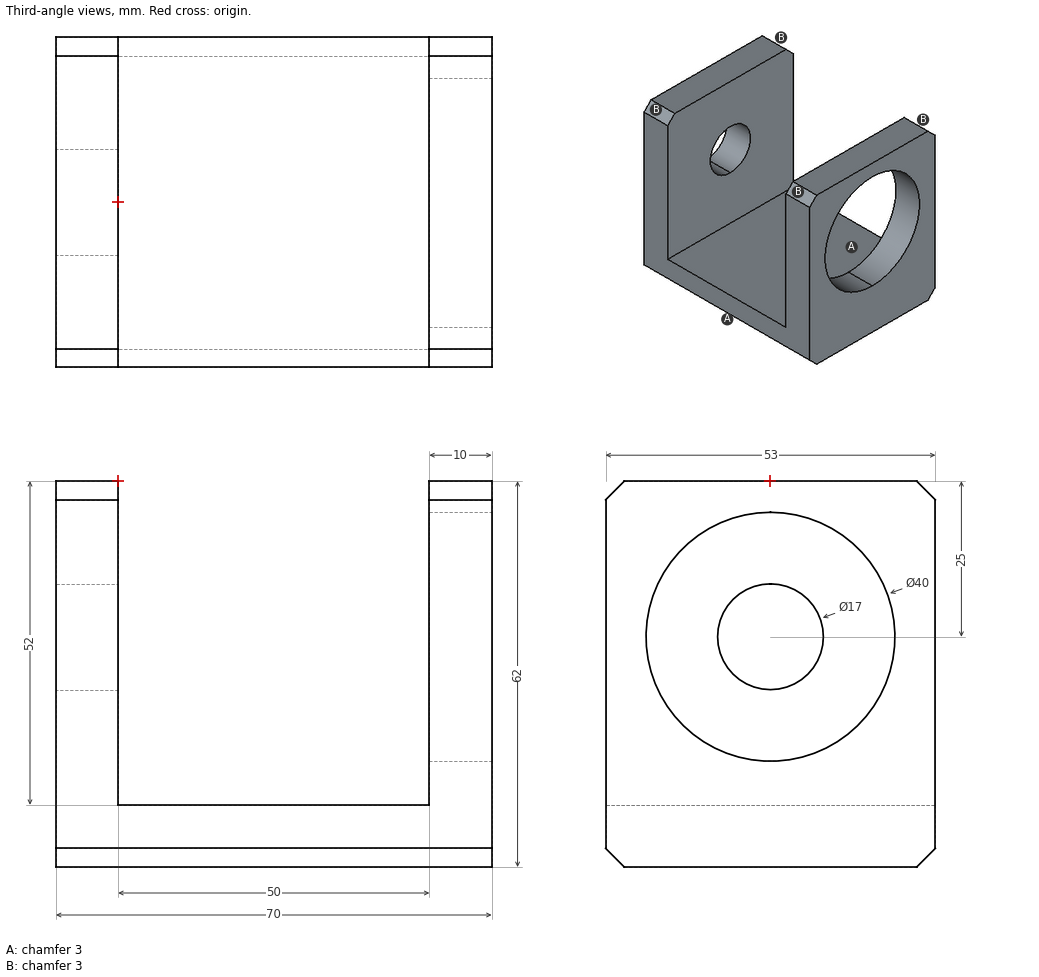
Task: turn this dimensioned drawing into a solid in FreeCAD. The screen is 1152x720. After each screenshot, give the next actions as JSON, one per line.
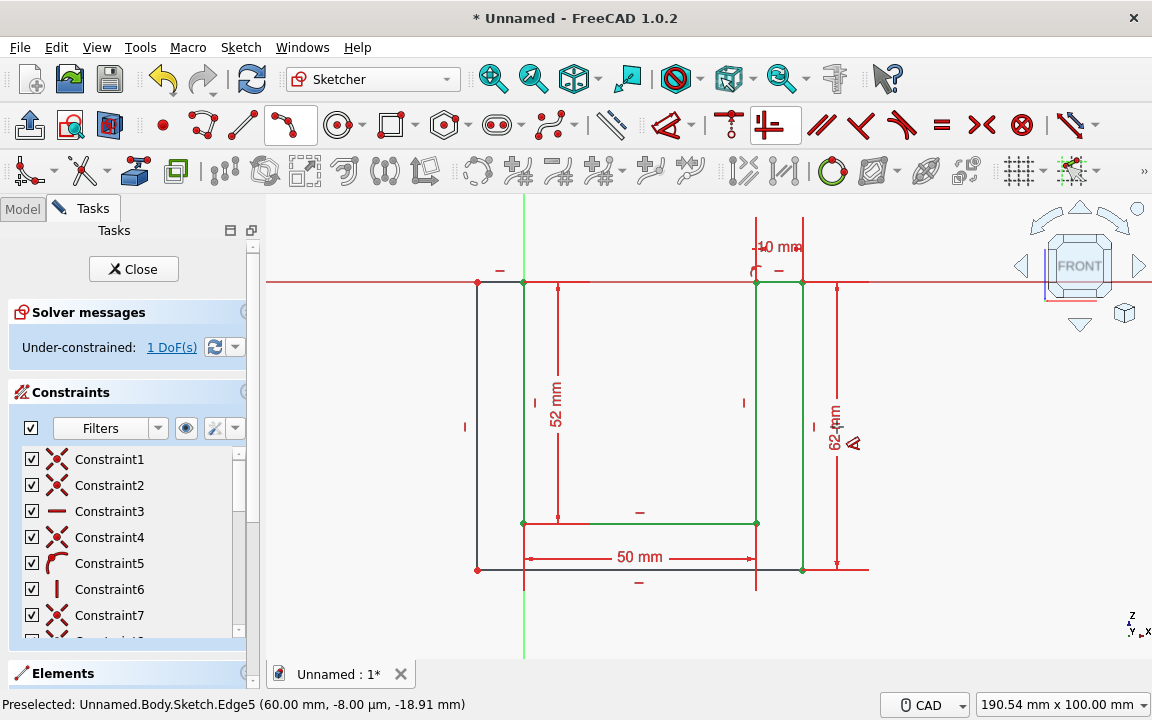
{"action": "left_click", "coordinate": [705, 570]}
{"action": "left_click", "coordinate": [640, 604]}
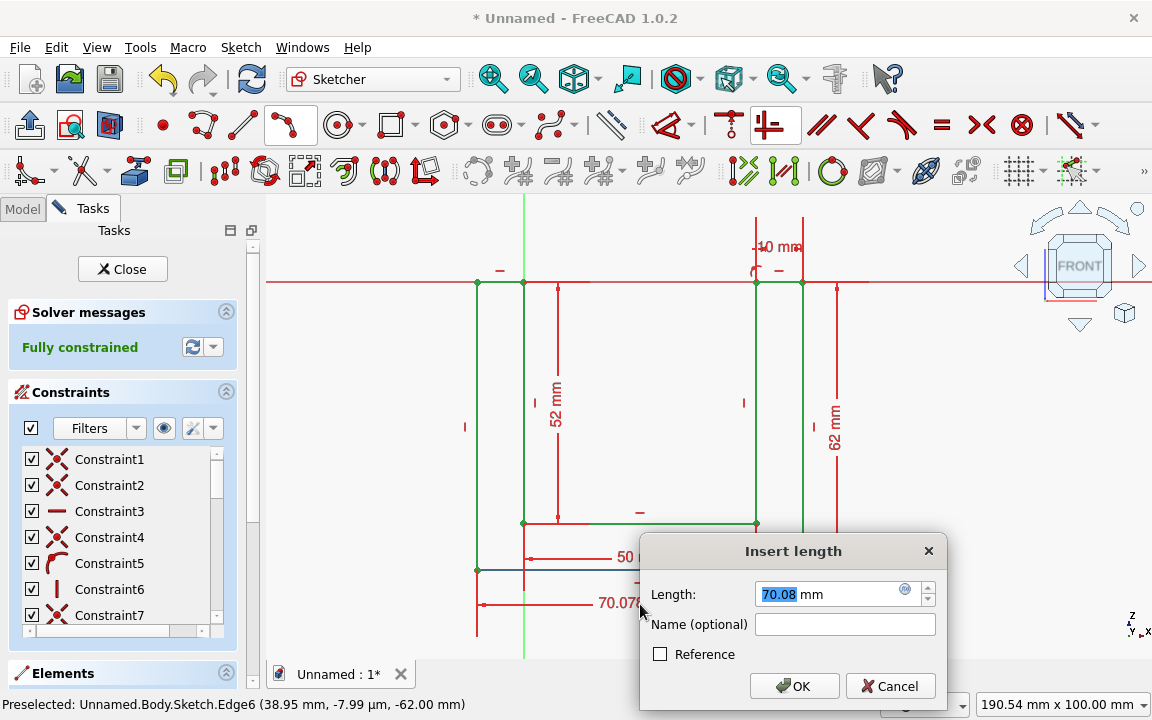
{"action": "type", "text": "70"}
{"action": "key", "text": "Return"}
{"action": "key", "text": "Escape"}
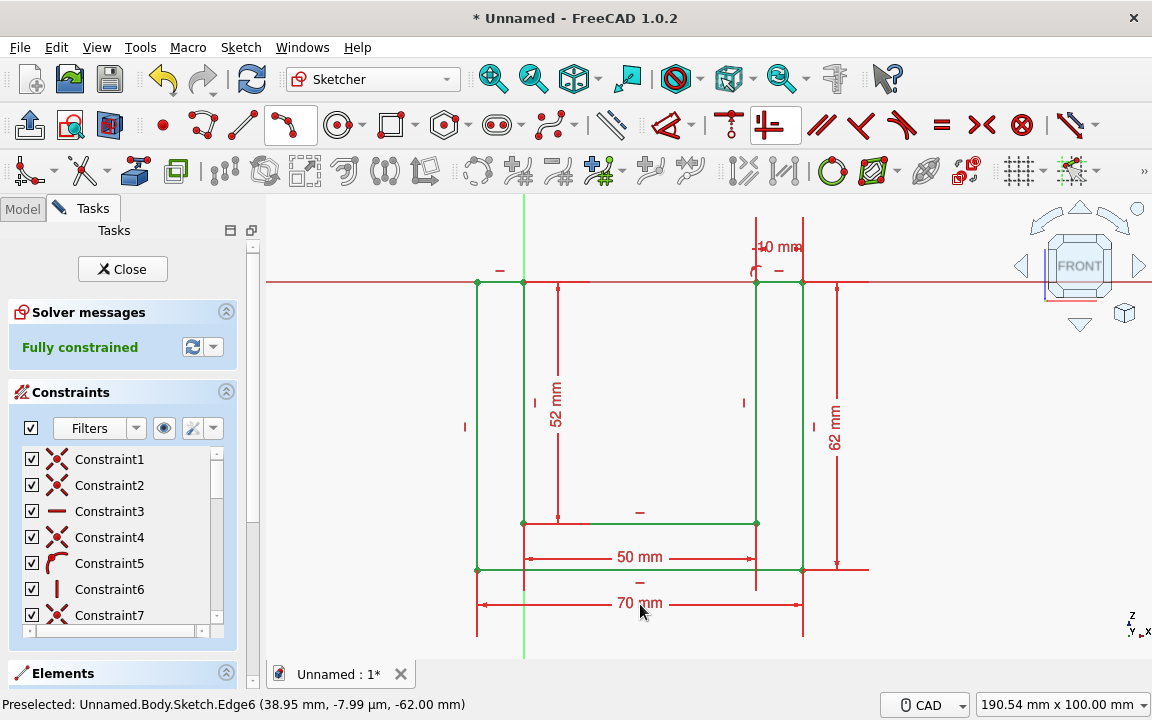
{"action": "left_click", "coordinate": [123, 269]}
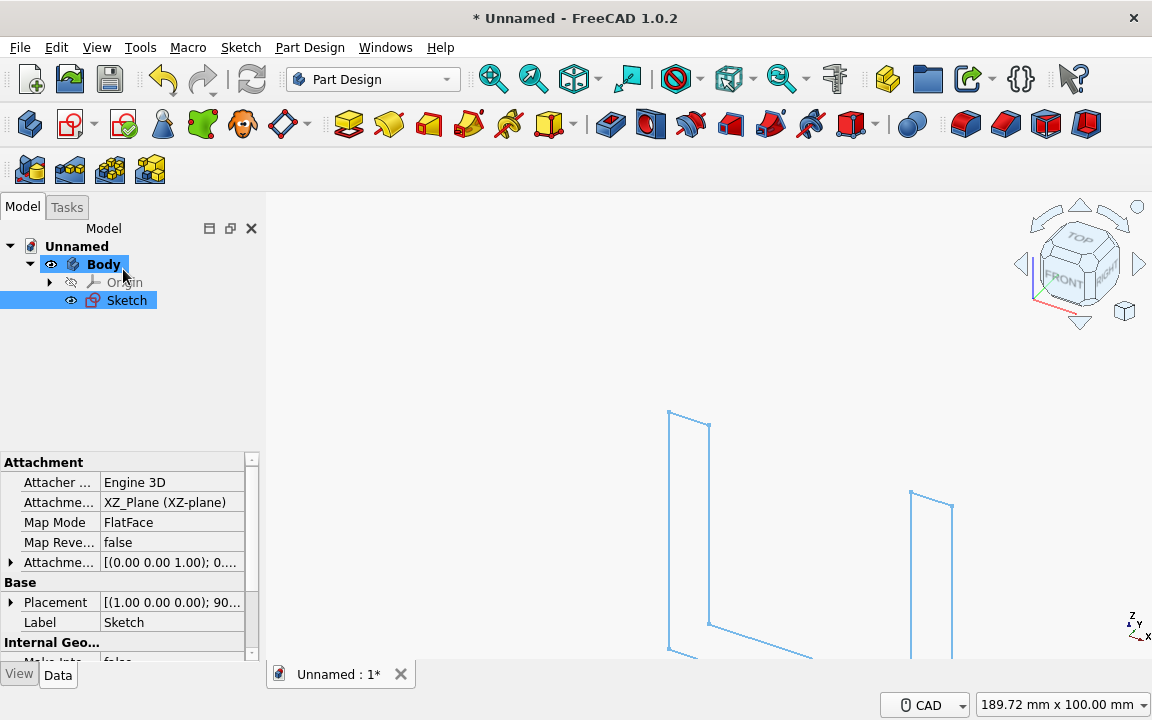
{"action": "left_click", "coordinate": [350, 124]}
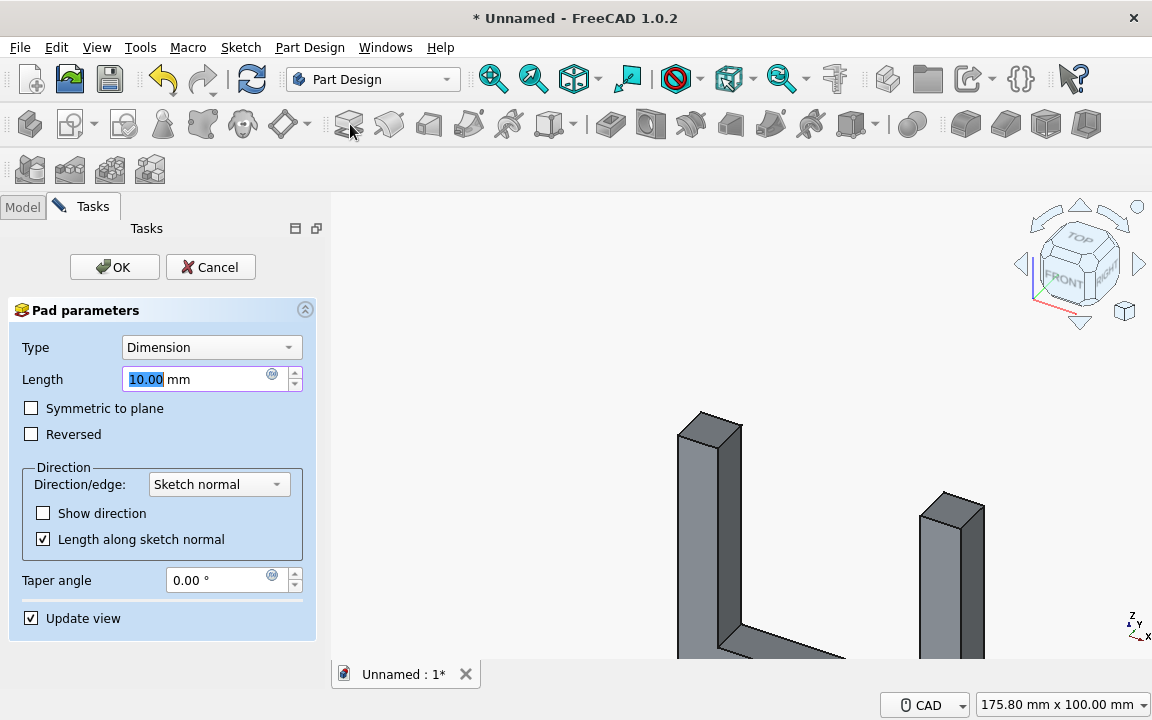
{"action": "type", "text": "53"}
{"action": "key", "text": "Tab"}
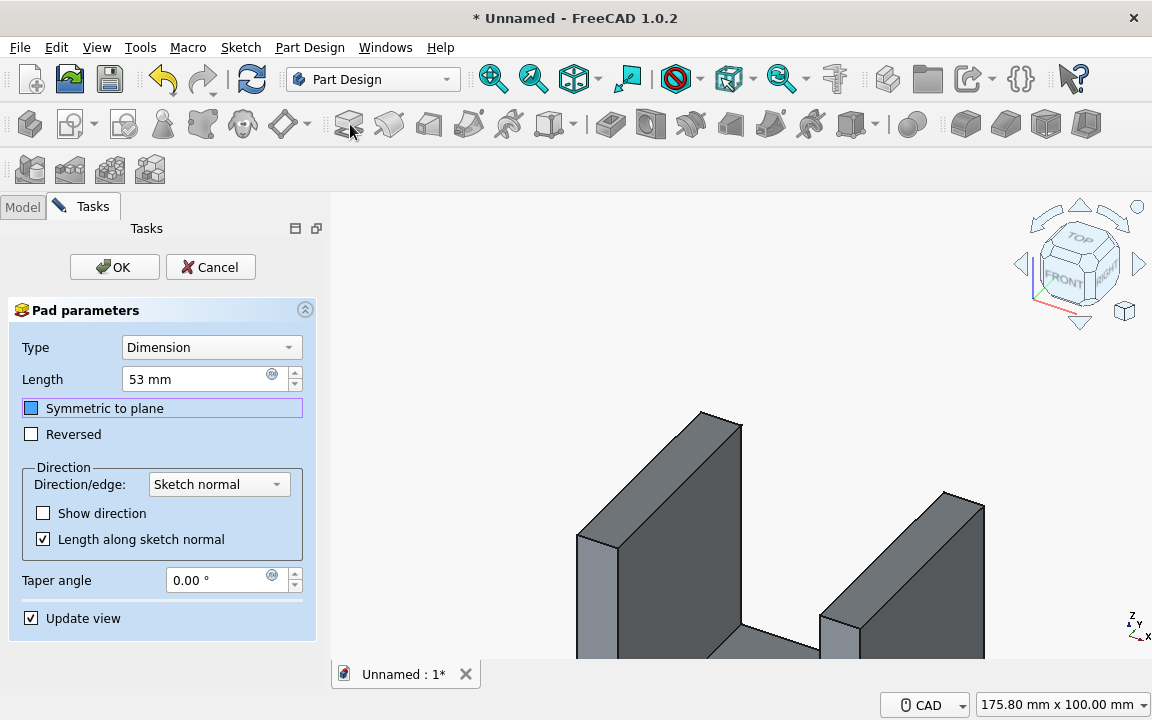
{"action": "left_click", "coordinate": [30, 408]}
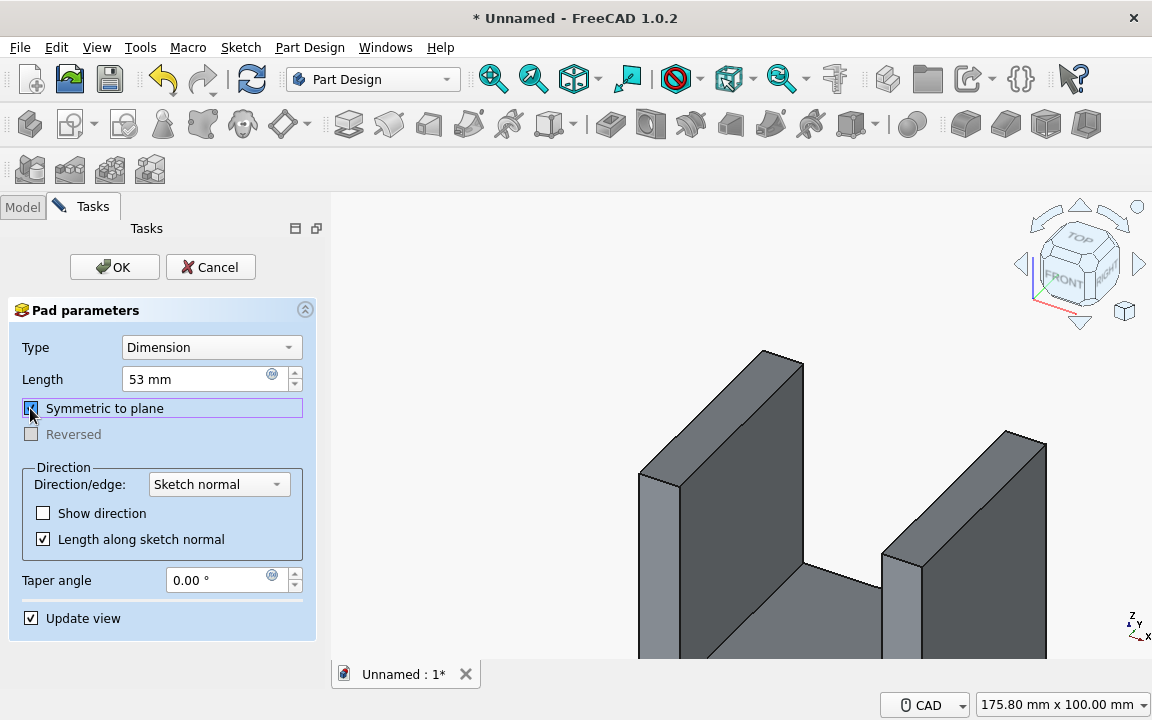
{"action": "left_click", "coordinate": [115, 267]}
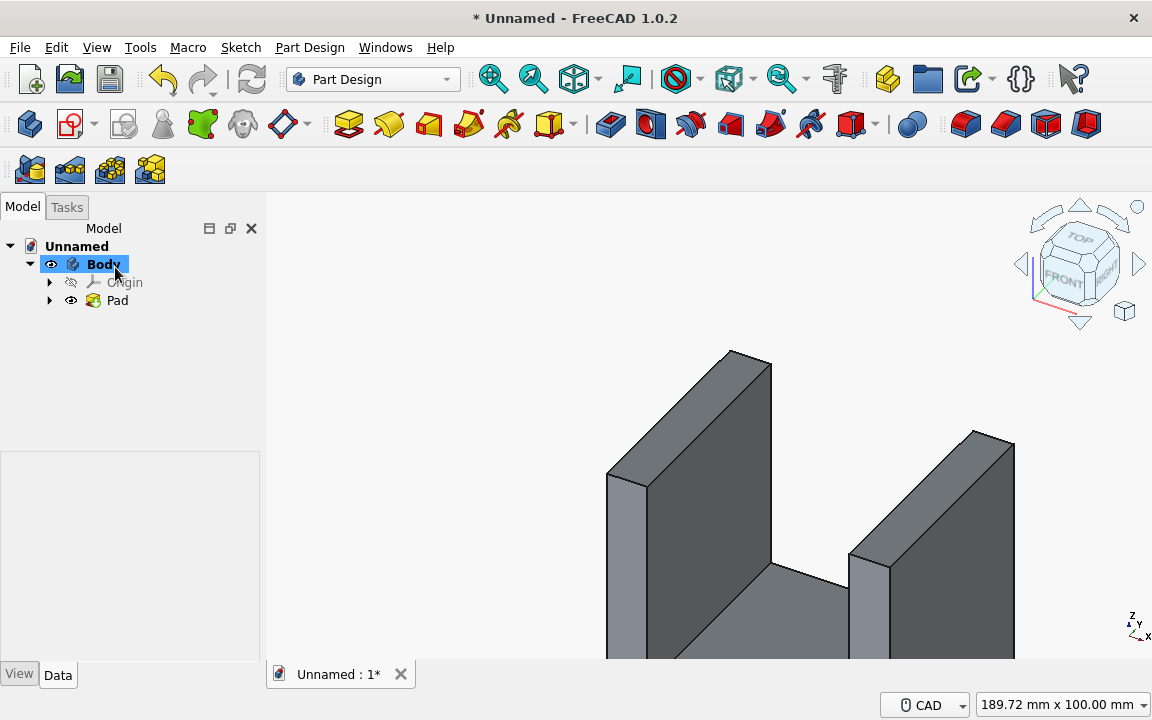
{"action": "key", "text": "v f"}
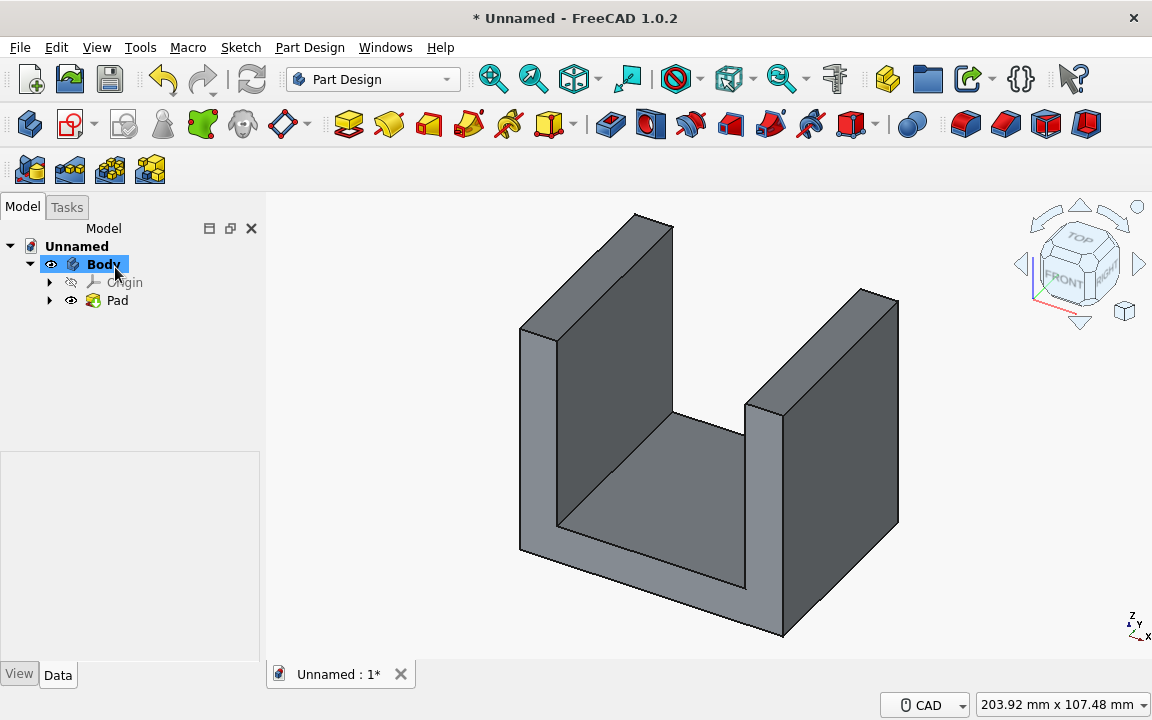
{"action": "key", "text": "6"}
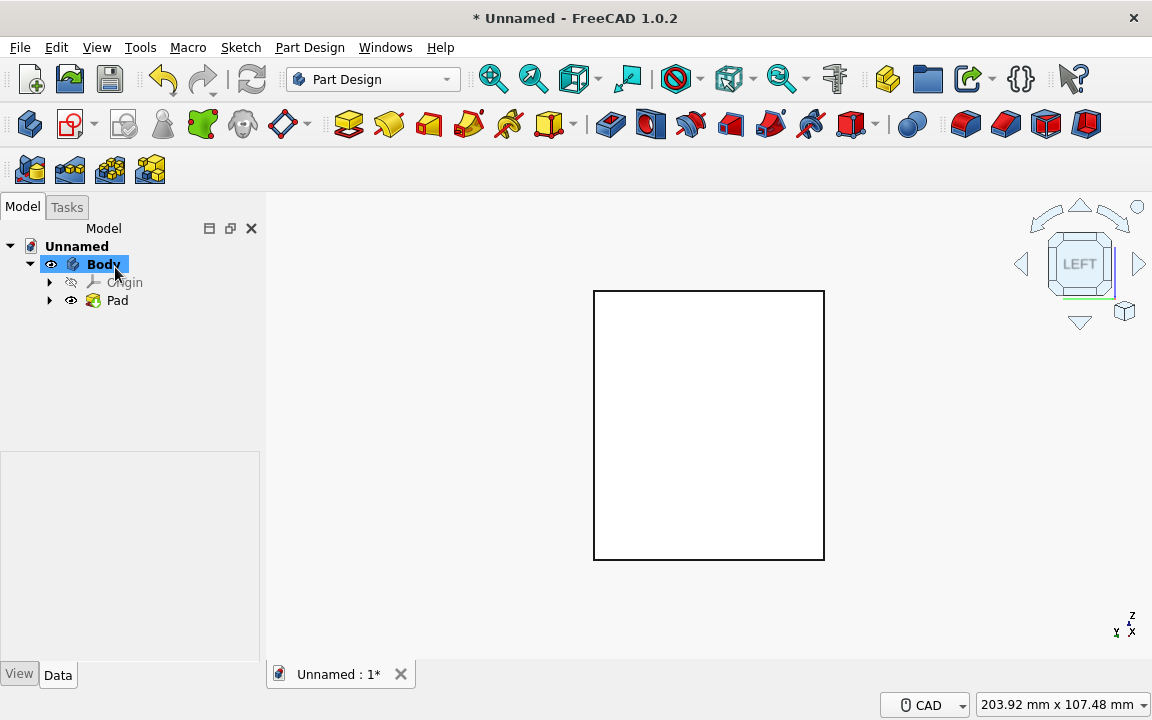
{"action": "left_click", "coordinate": [709, 424]}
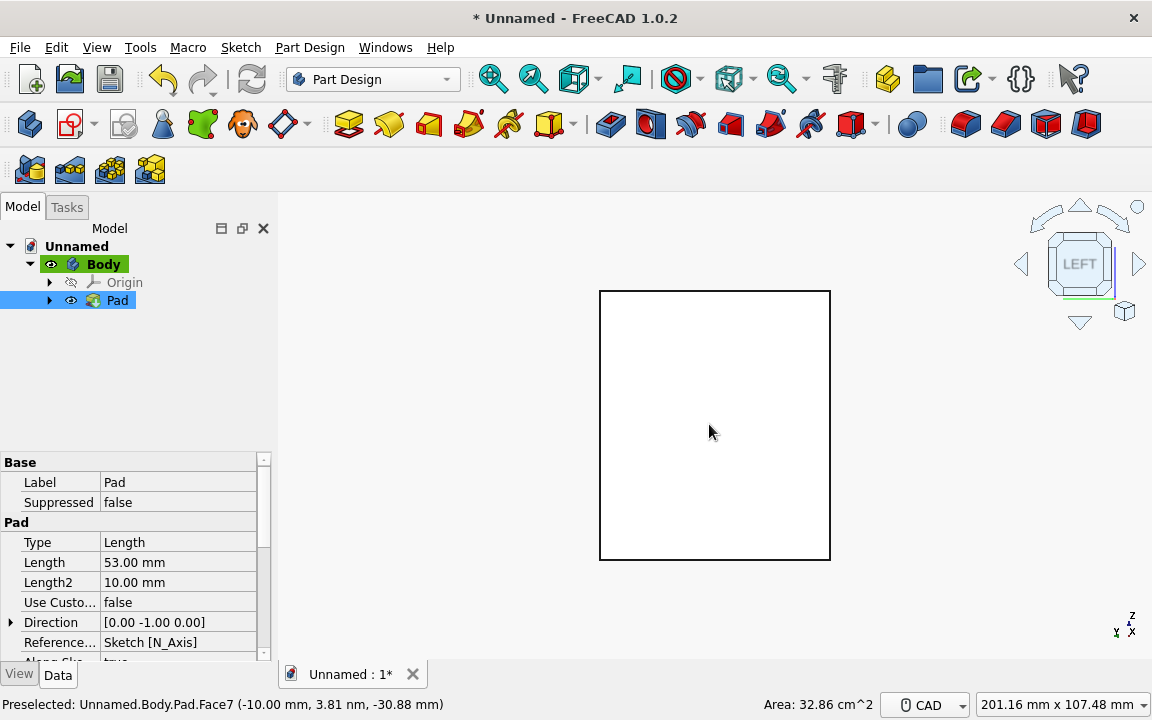
{"action": "left_click", "coordinate": [70, 124]}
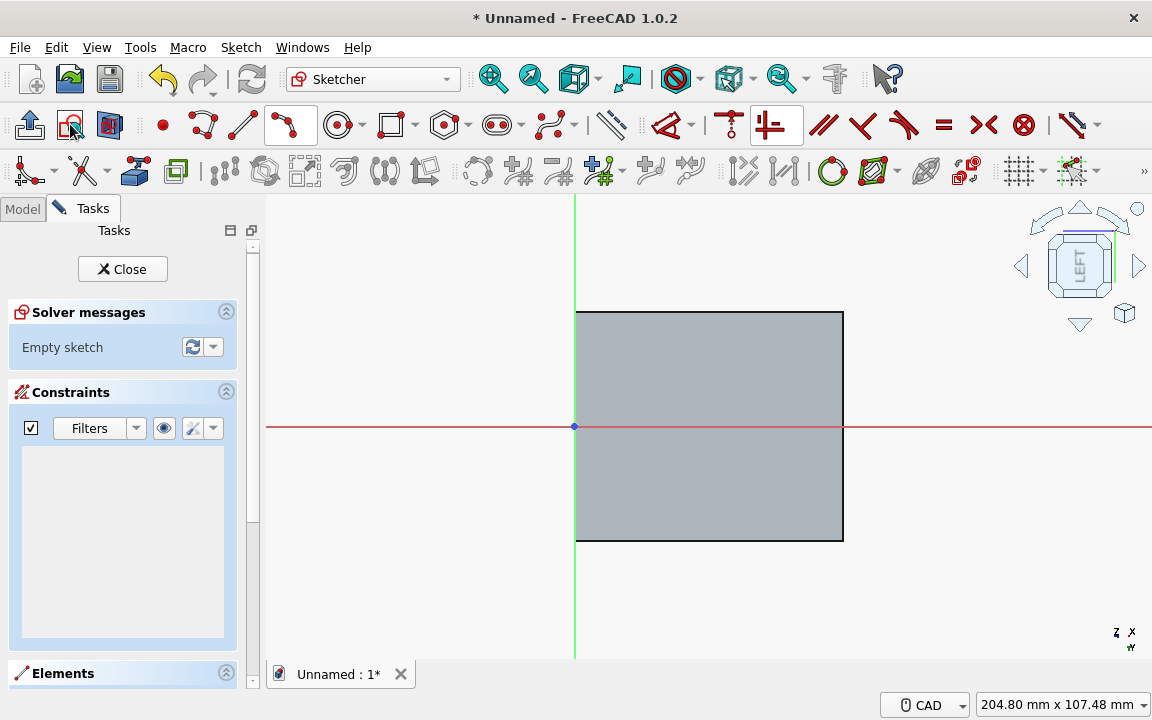
{"action": "scroll", "coordinate": [650, 426], "scroll_direction": "up", "scroll_amount": 6}